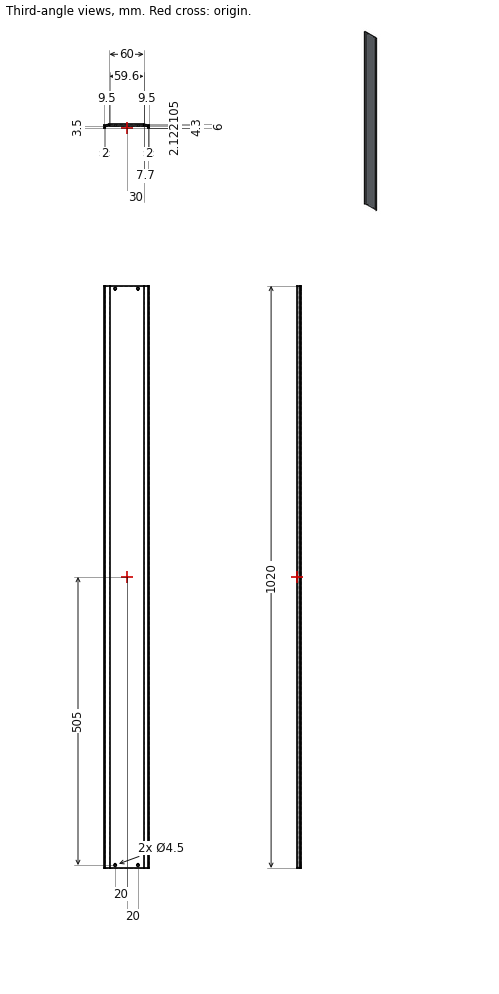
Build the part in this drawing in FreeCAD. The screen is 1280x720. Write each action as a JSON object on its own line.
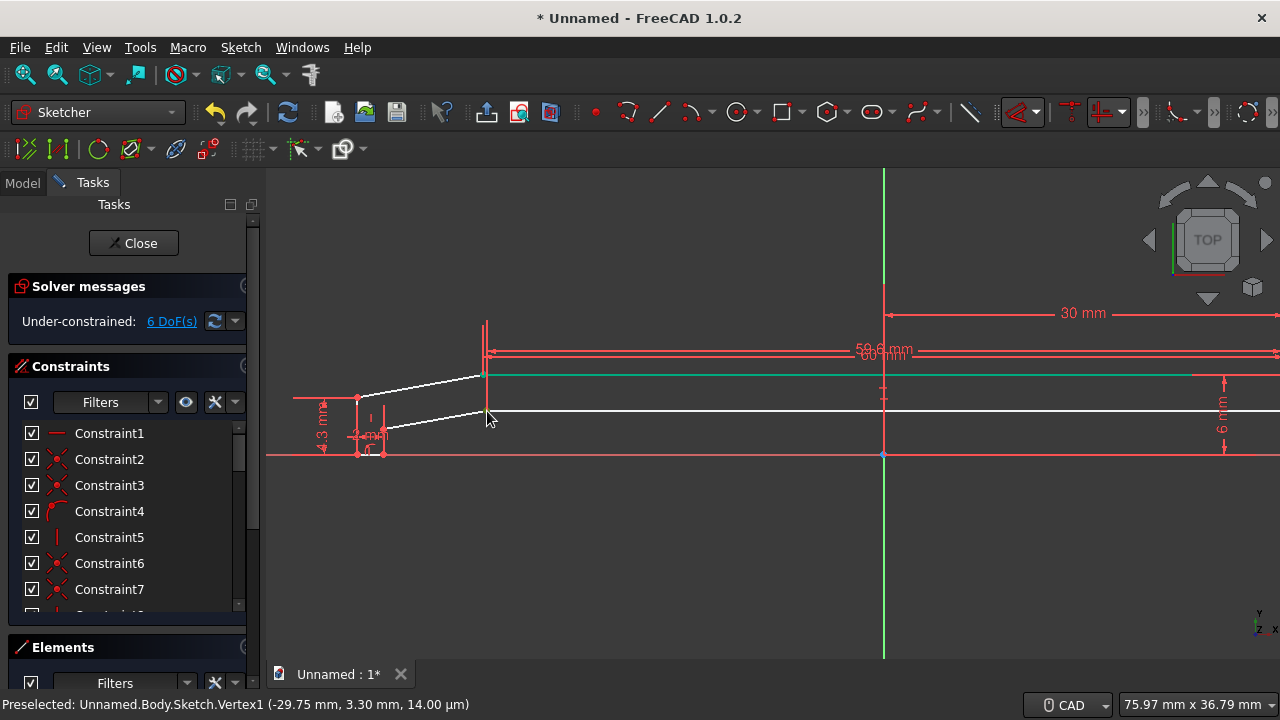
{"action": "key", "text": "i"}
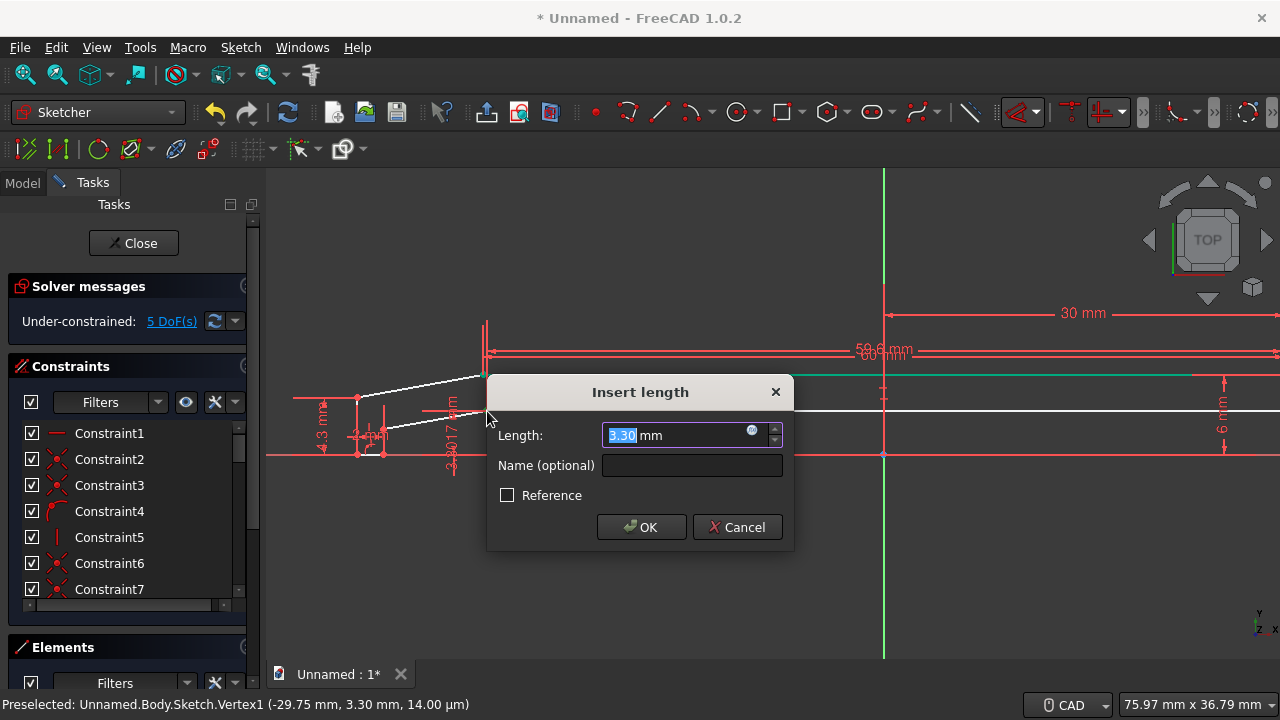
{"action": "type", "text": "3.5"}
{"action": "key", "text": "Return"}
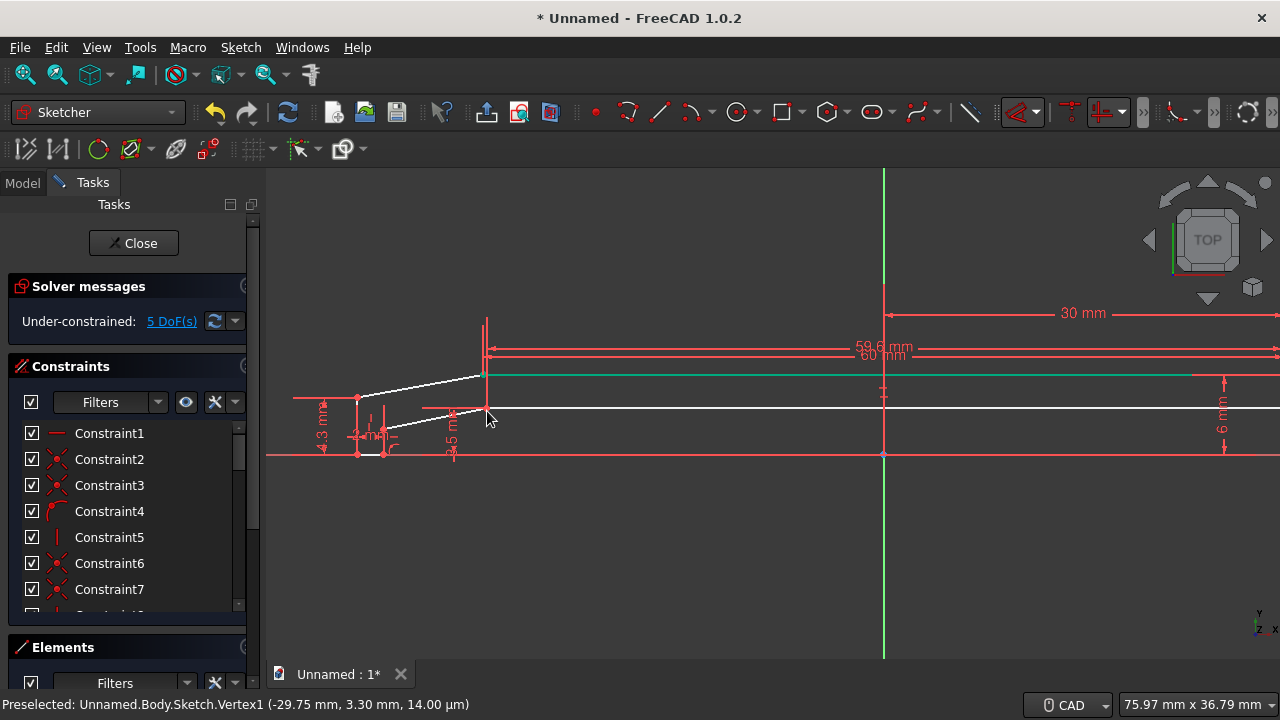
{"action": "scroll", "coordinate": [487, 412], "scroll_direction": "down", "scroll_amount": 3}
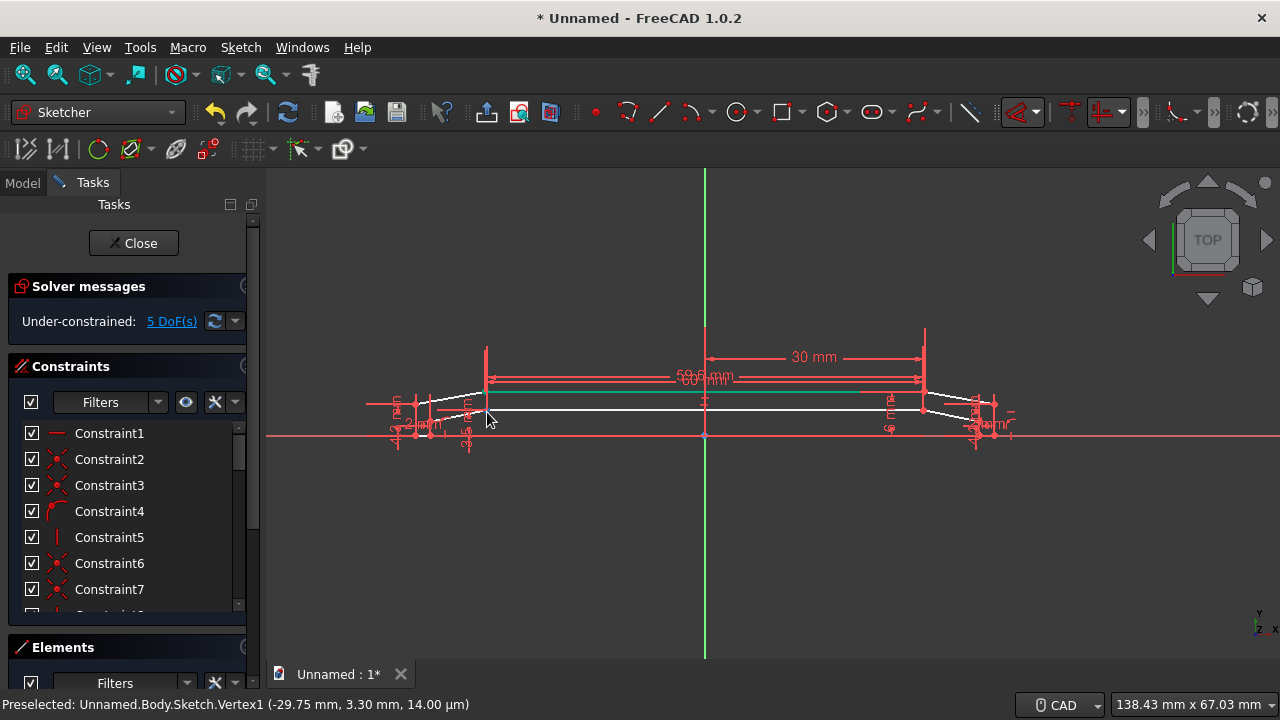
{"action": "left_click", "coordinate": [940, 414]}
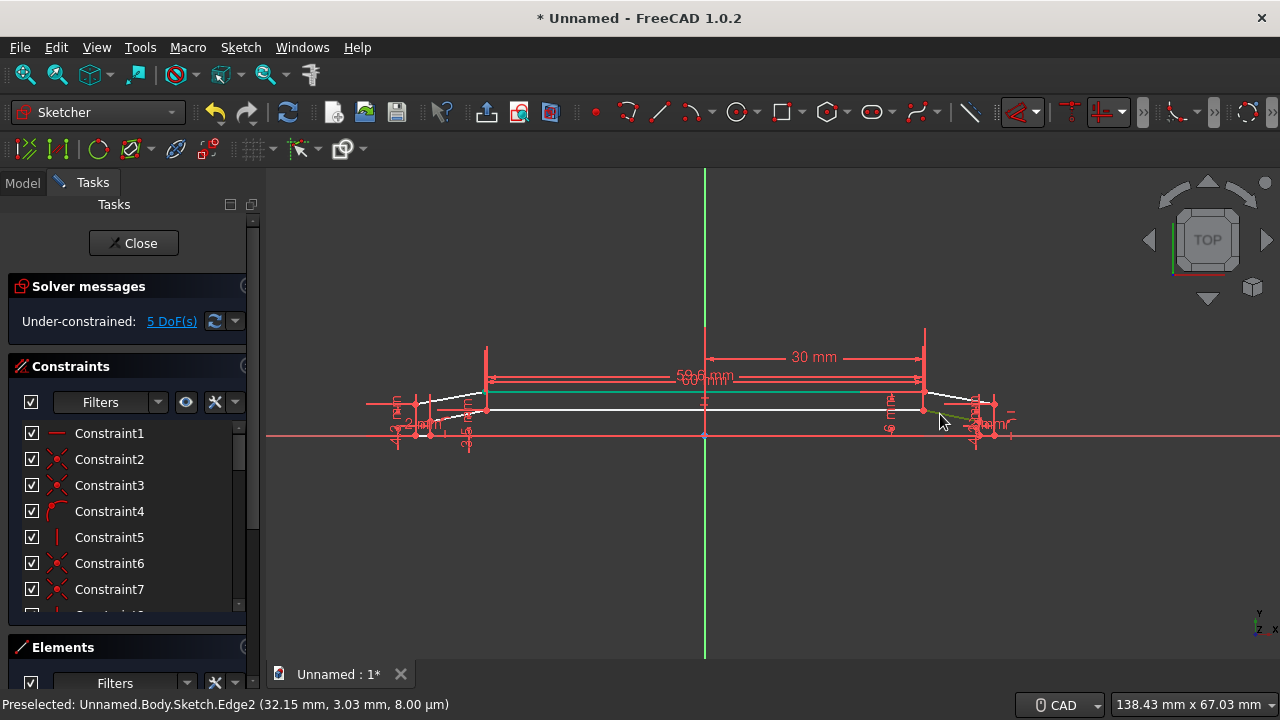
{"action": "left_click", "coordinate": [1038, 112]}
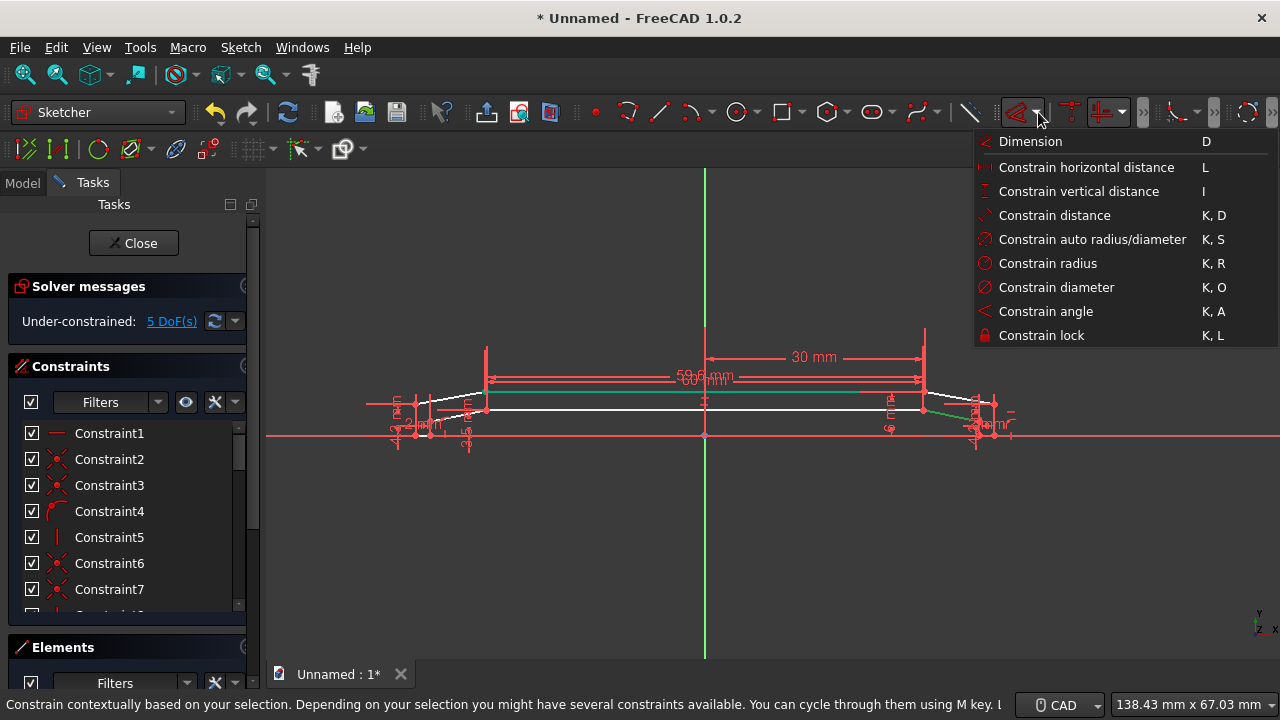
{"action": "left_click", "coordinate": [1126, 167]}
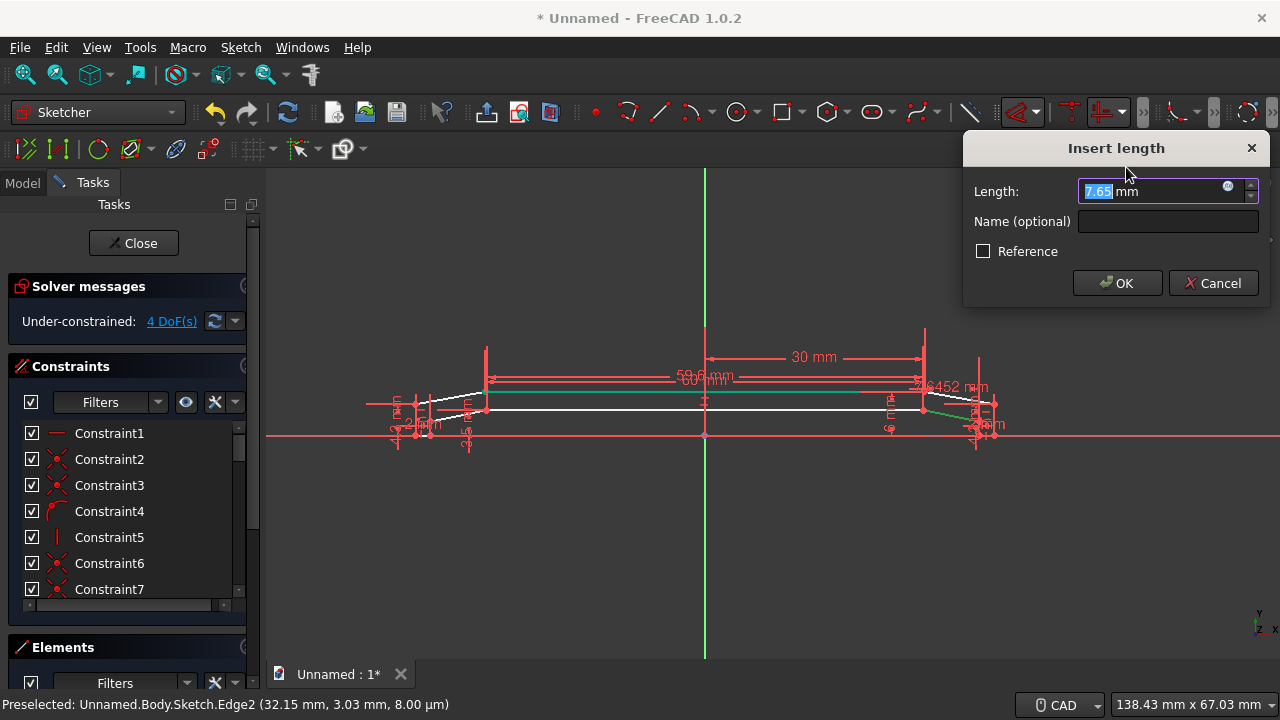
{"action": "type", "text": "7.7"}
{"action": "key", "text": "Return"}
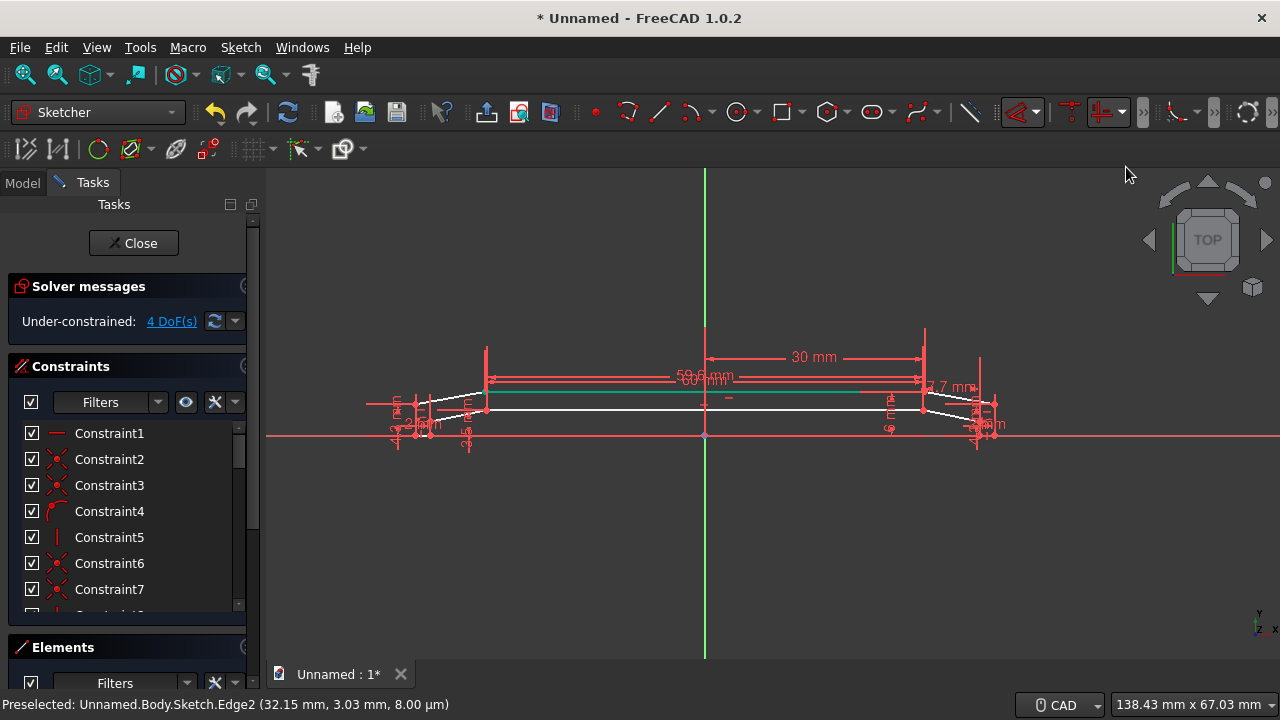
{"action": "left_click", "coordinate": [946, 396]}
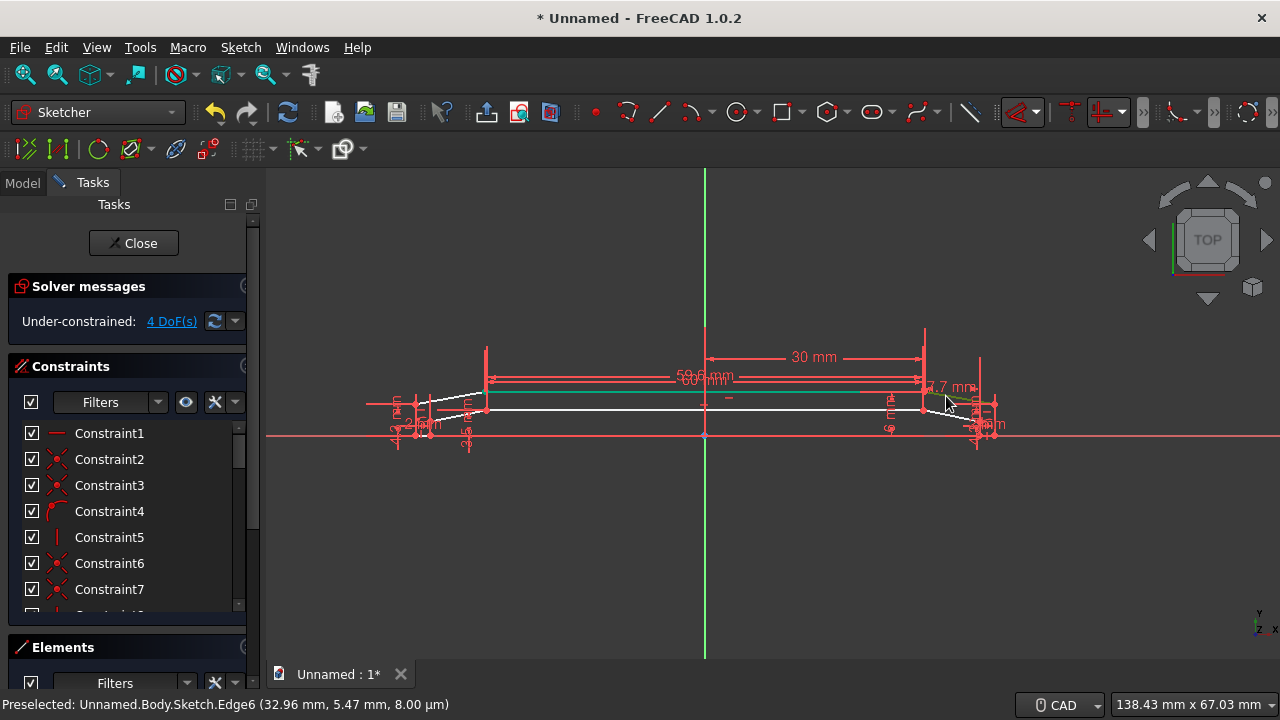
{"action": "key", "text": "l"}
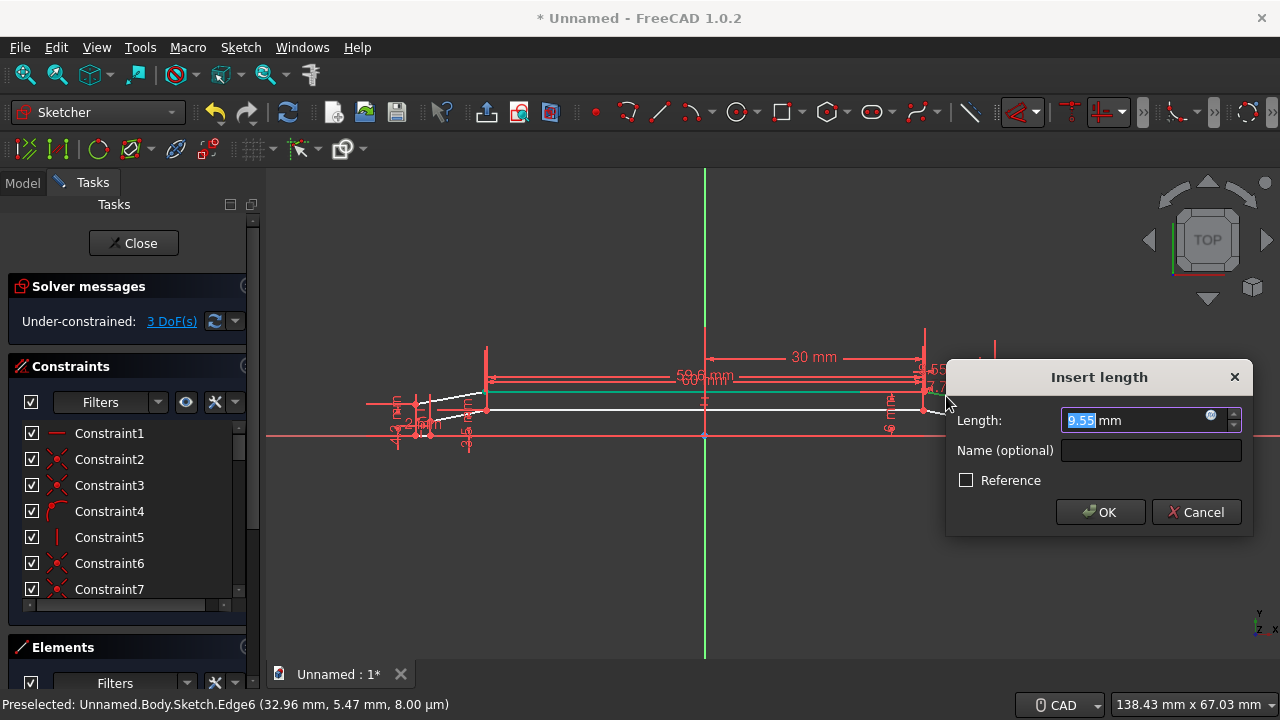
{"action": "type", "text": "9.5"}
{"action": "key", "text": "Return"}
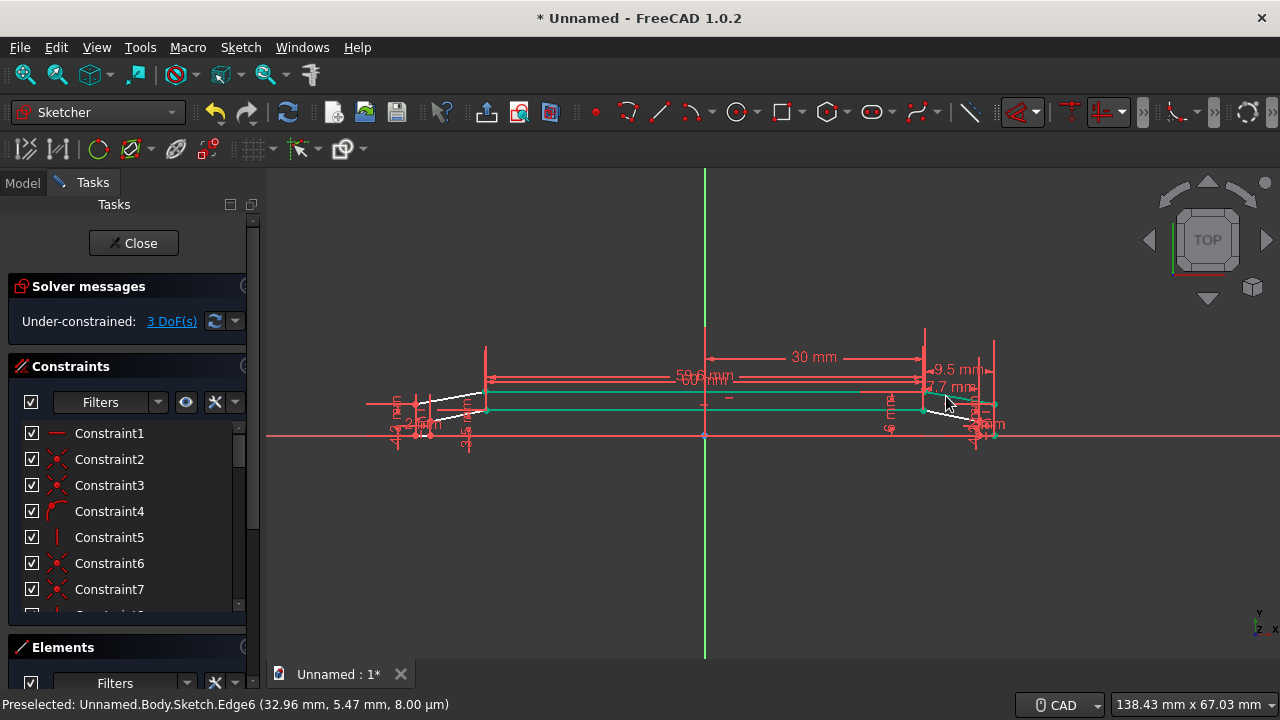
{"action": "left_click", "coordinate": [464, 396]}